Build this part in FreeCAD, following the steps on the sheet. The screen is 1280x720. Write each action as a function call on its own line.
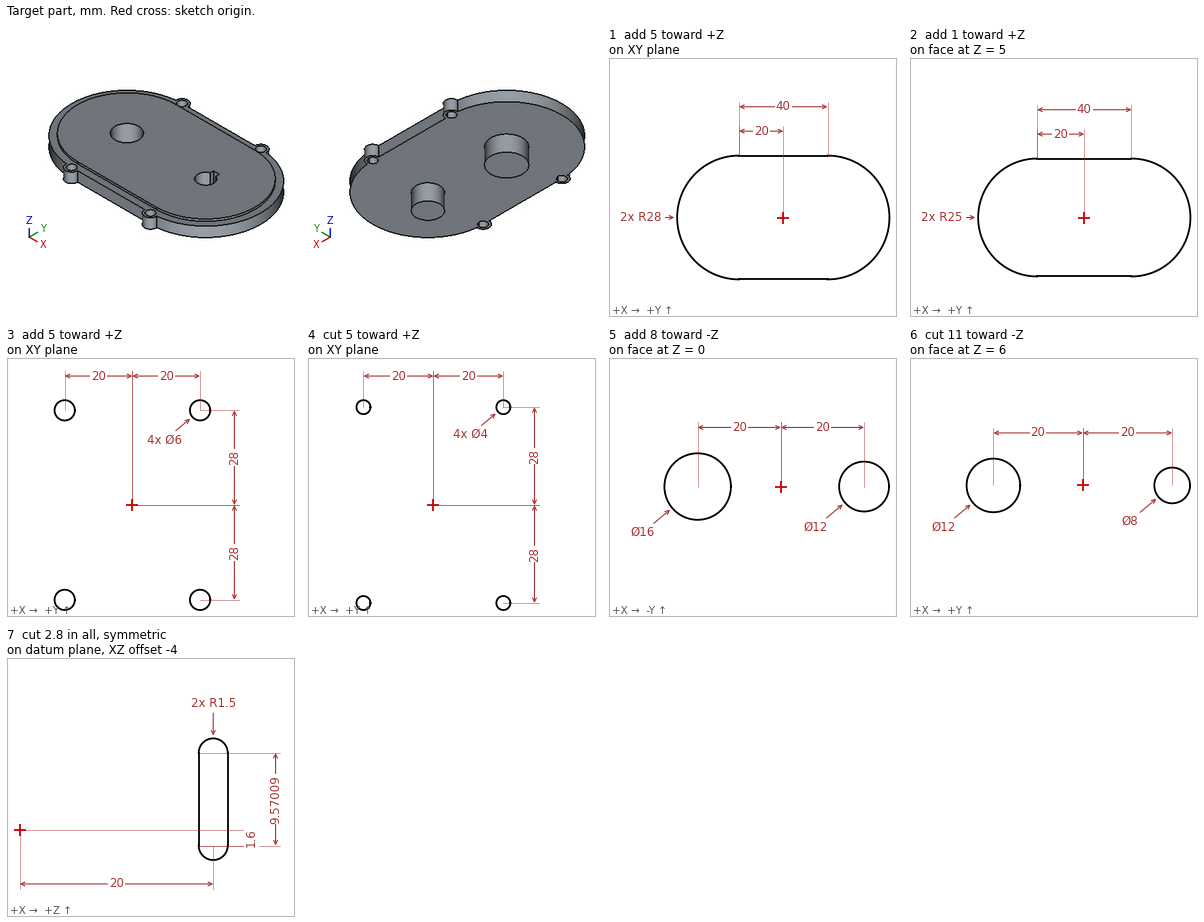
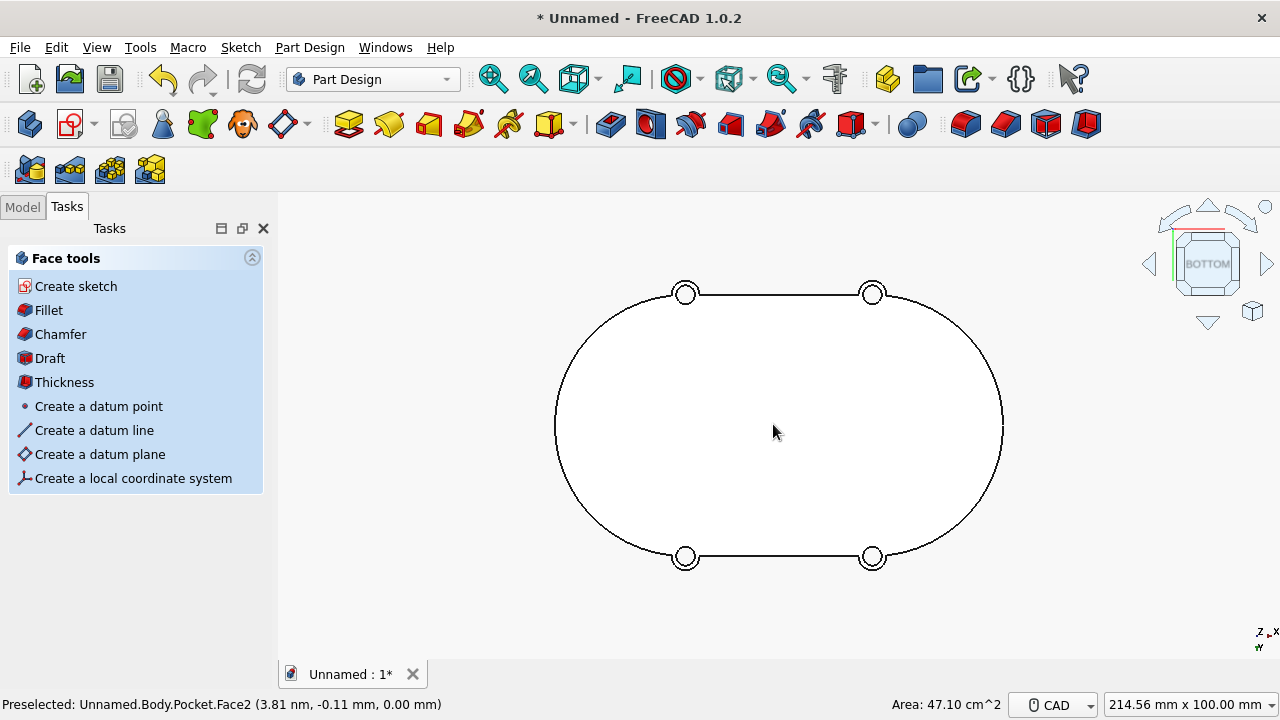
click(70, 124)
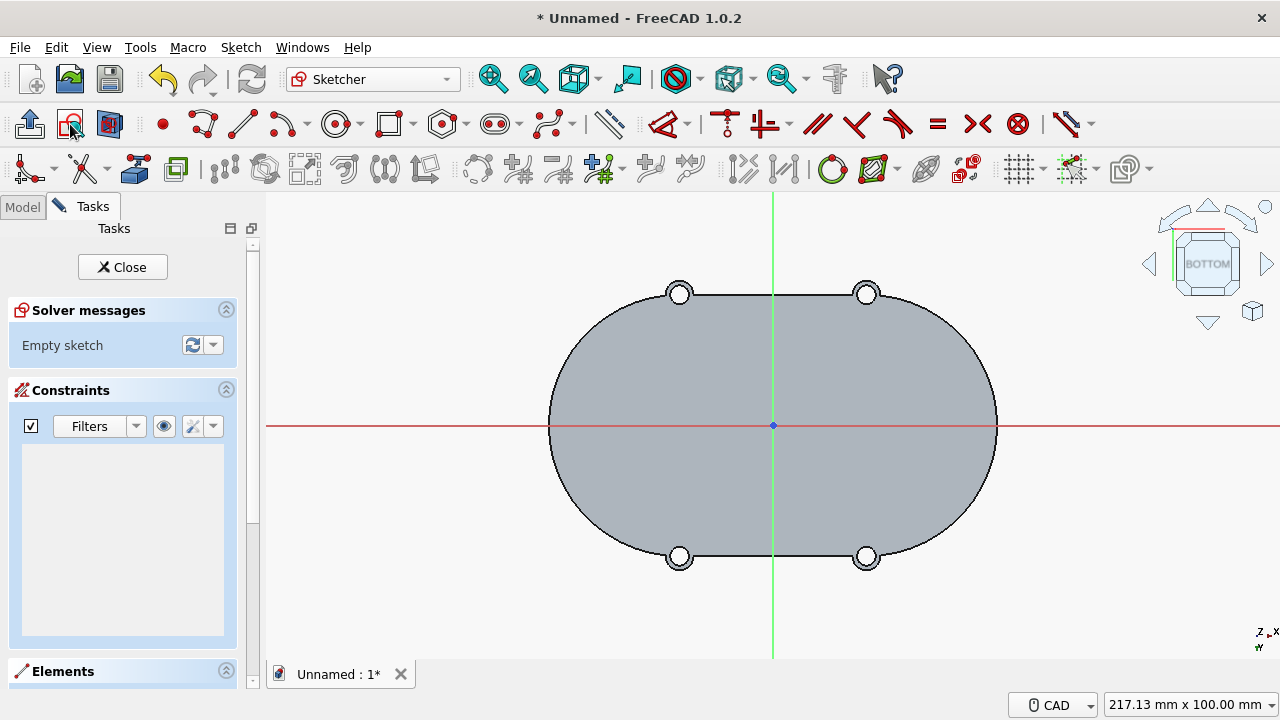
scroll(820, 426, up, 4)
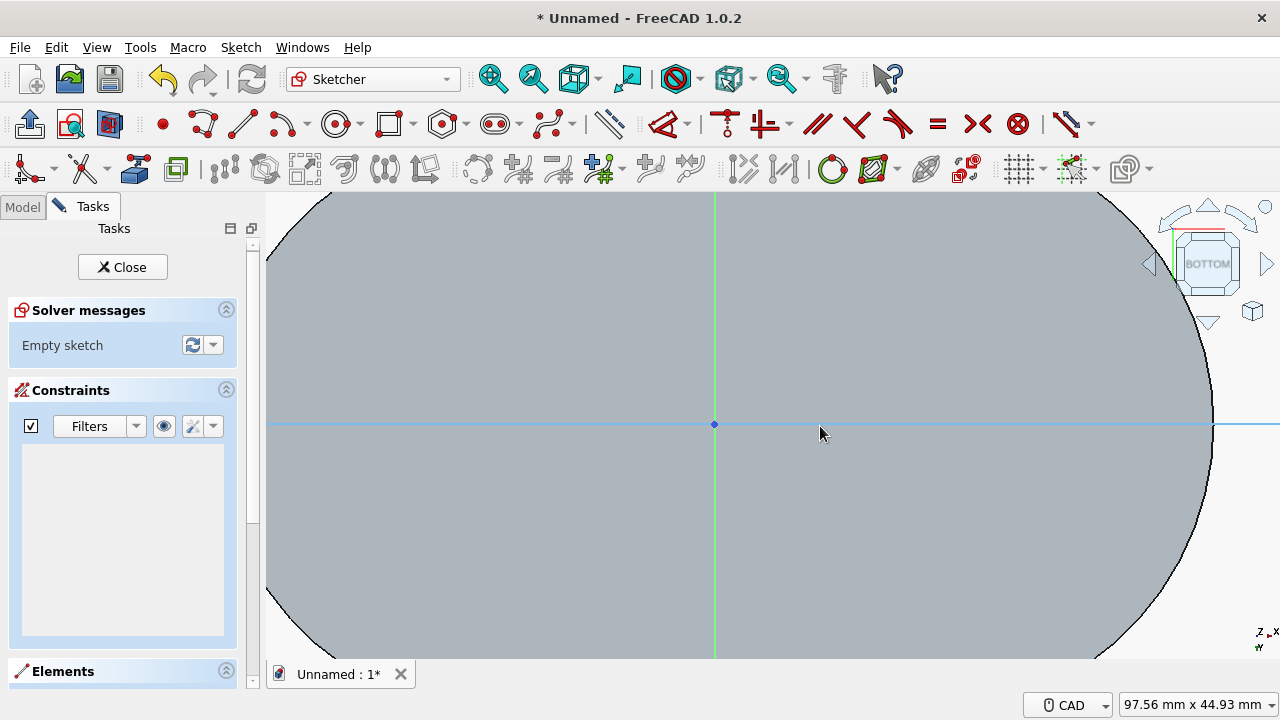
click(336, 124)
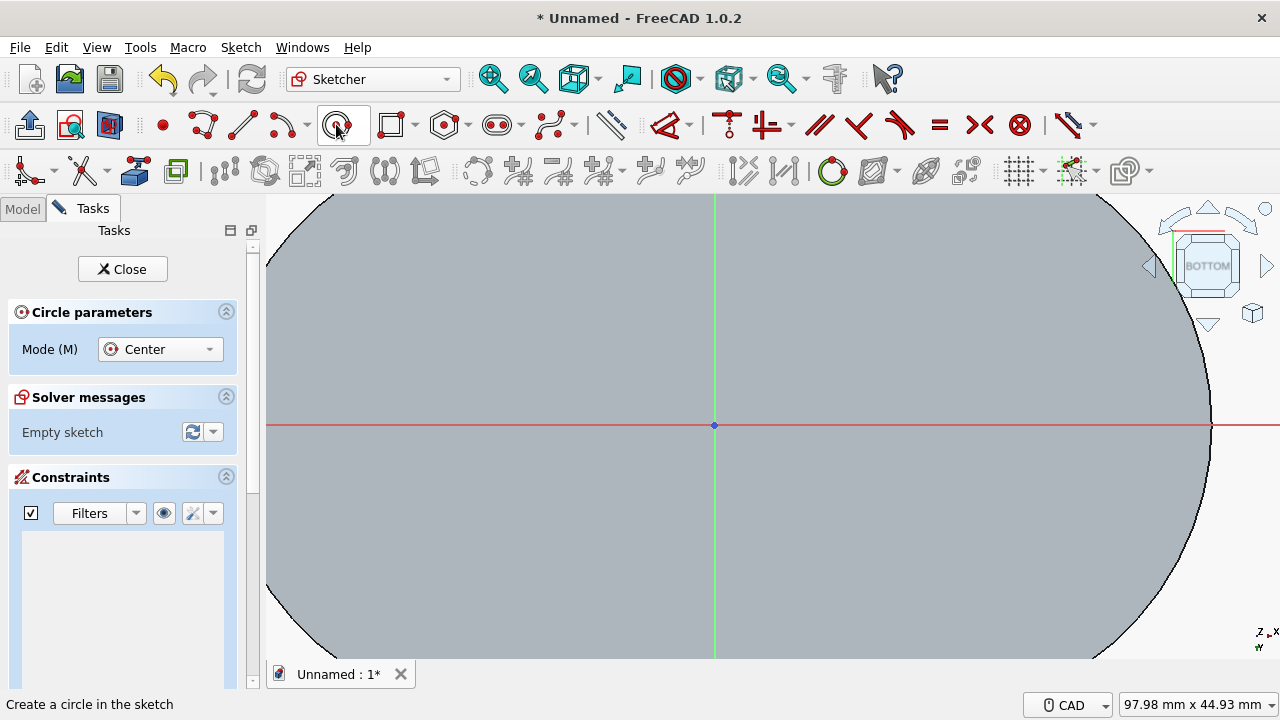
click(922, 425)
click(966, 381)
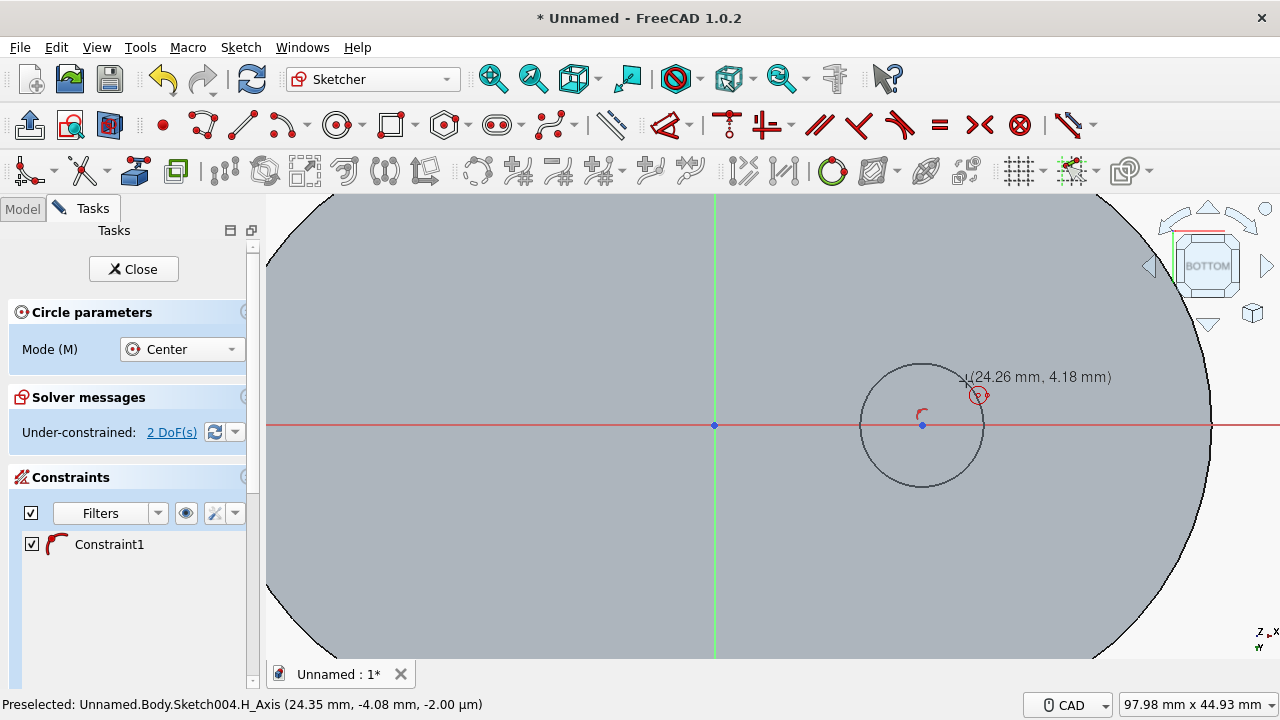
click(508, 425)
click(567, 367)
key(Escape)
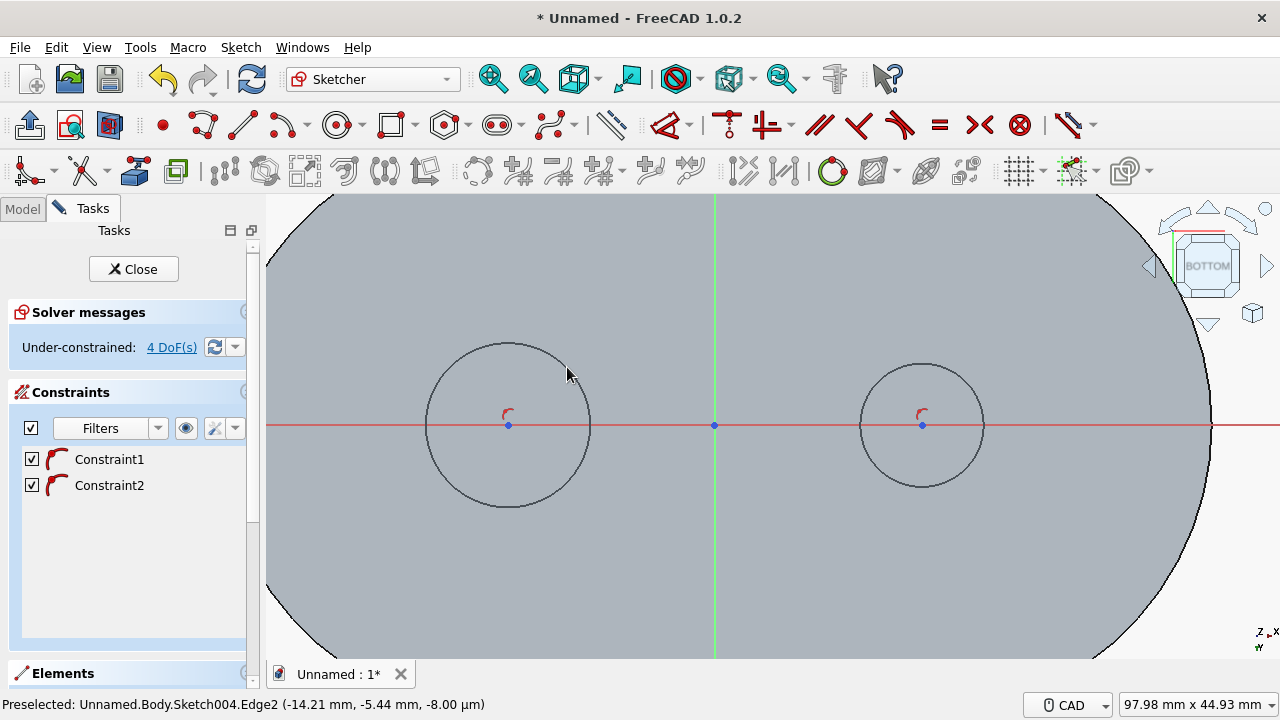
click(666, 126)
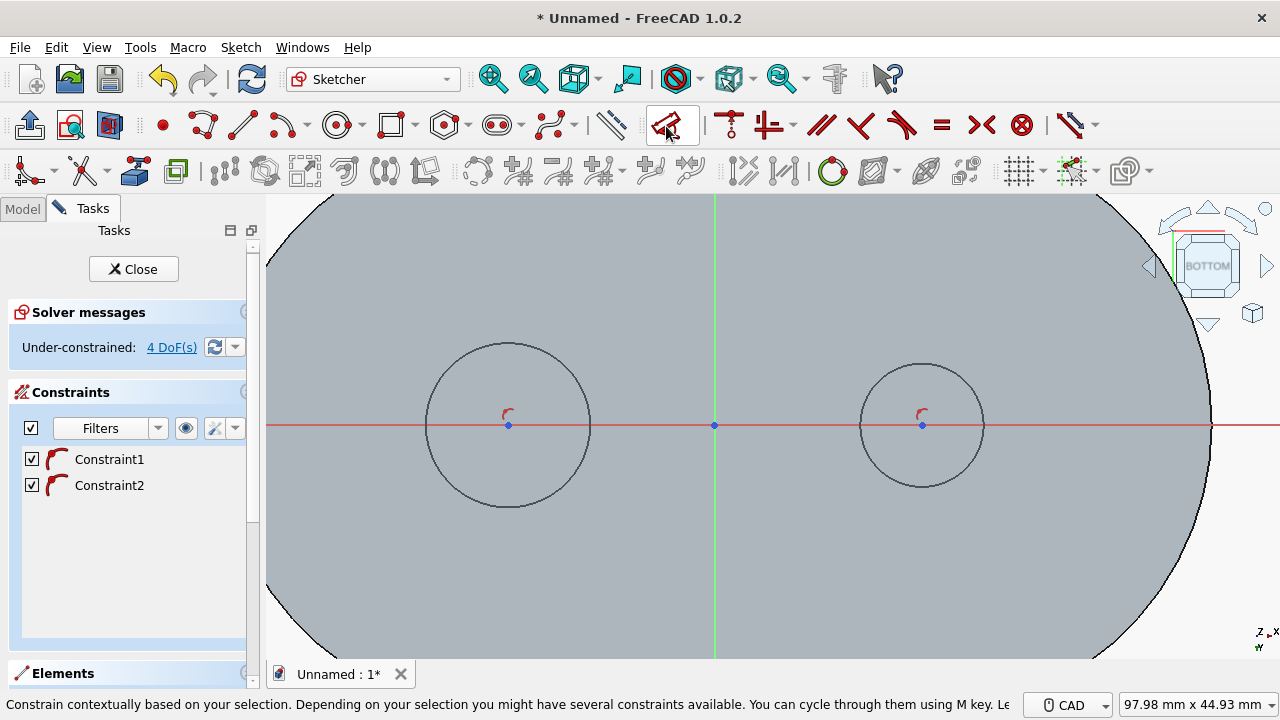
click(966, 382)
click(989, 360)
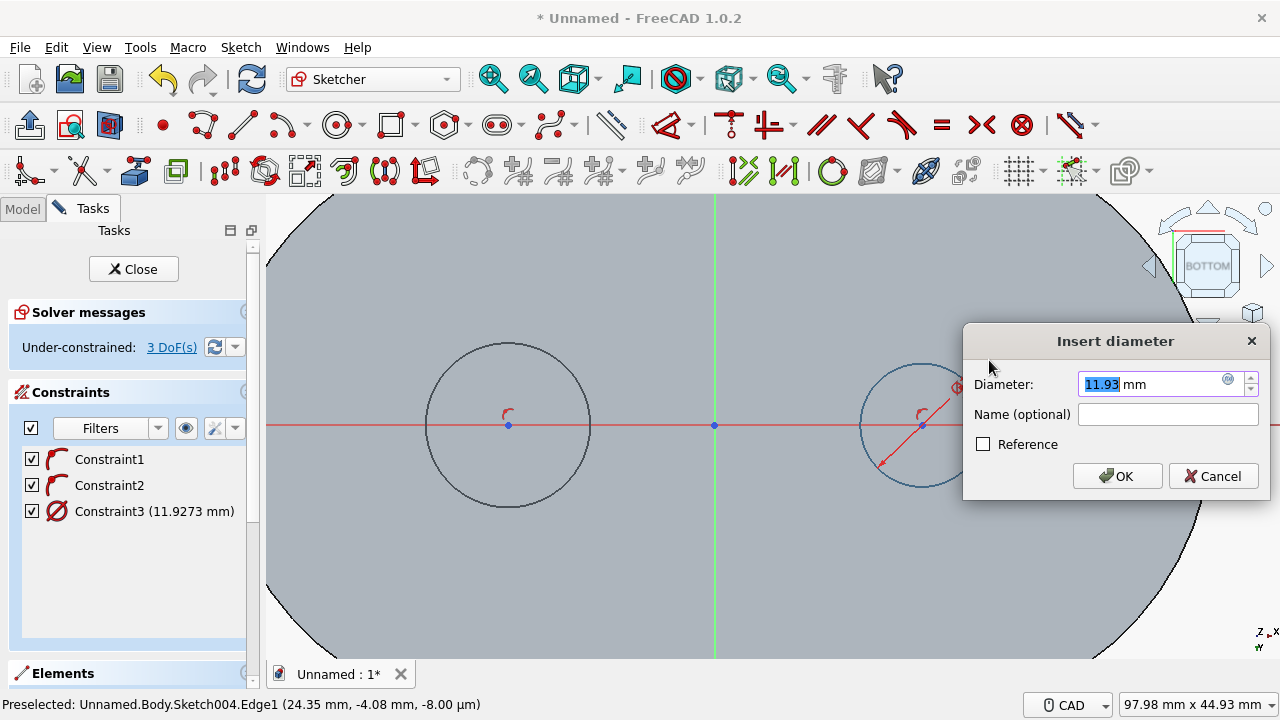
text(12)
key(Return)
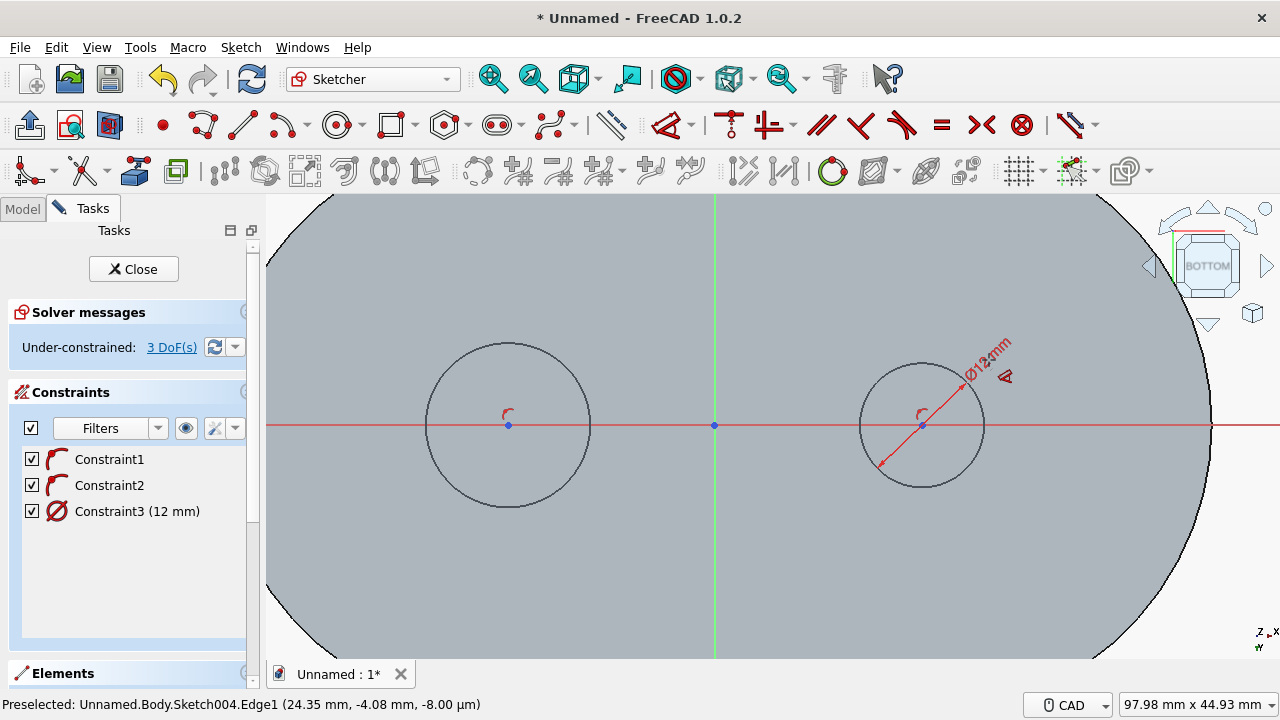
click(566, 367)
click(589, 344)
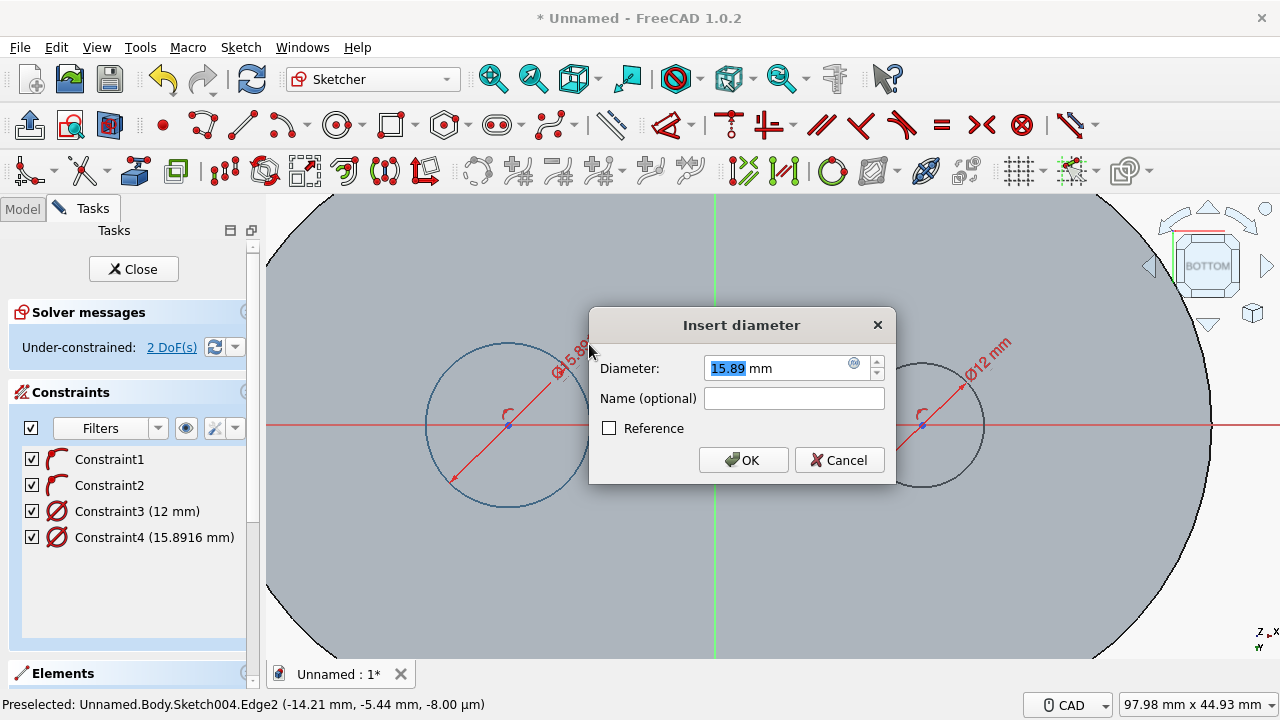
text(16)
key(Return)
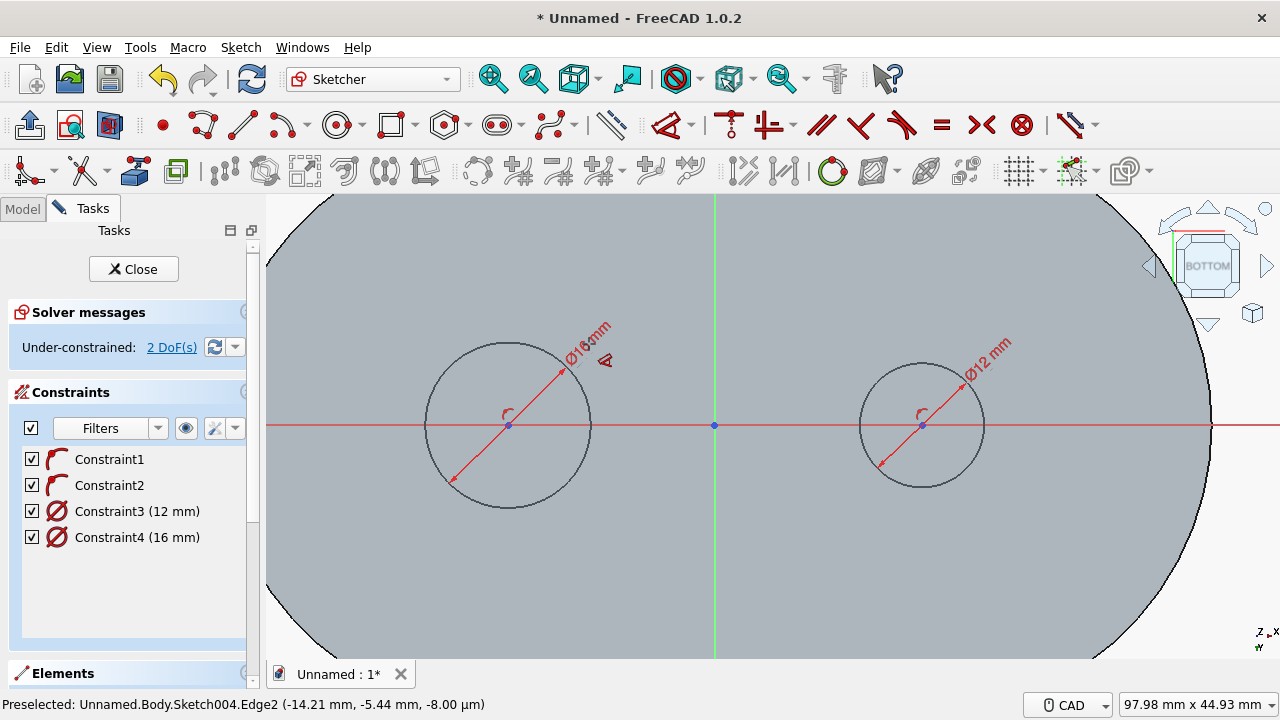
click(922, 425)
click(818, 459)